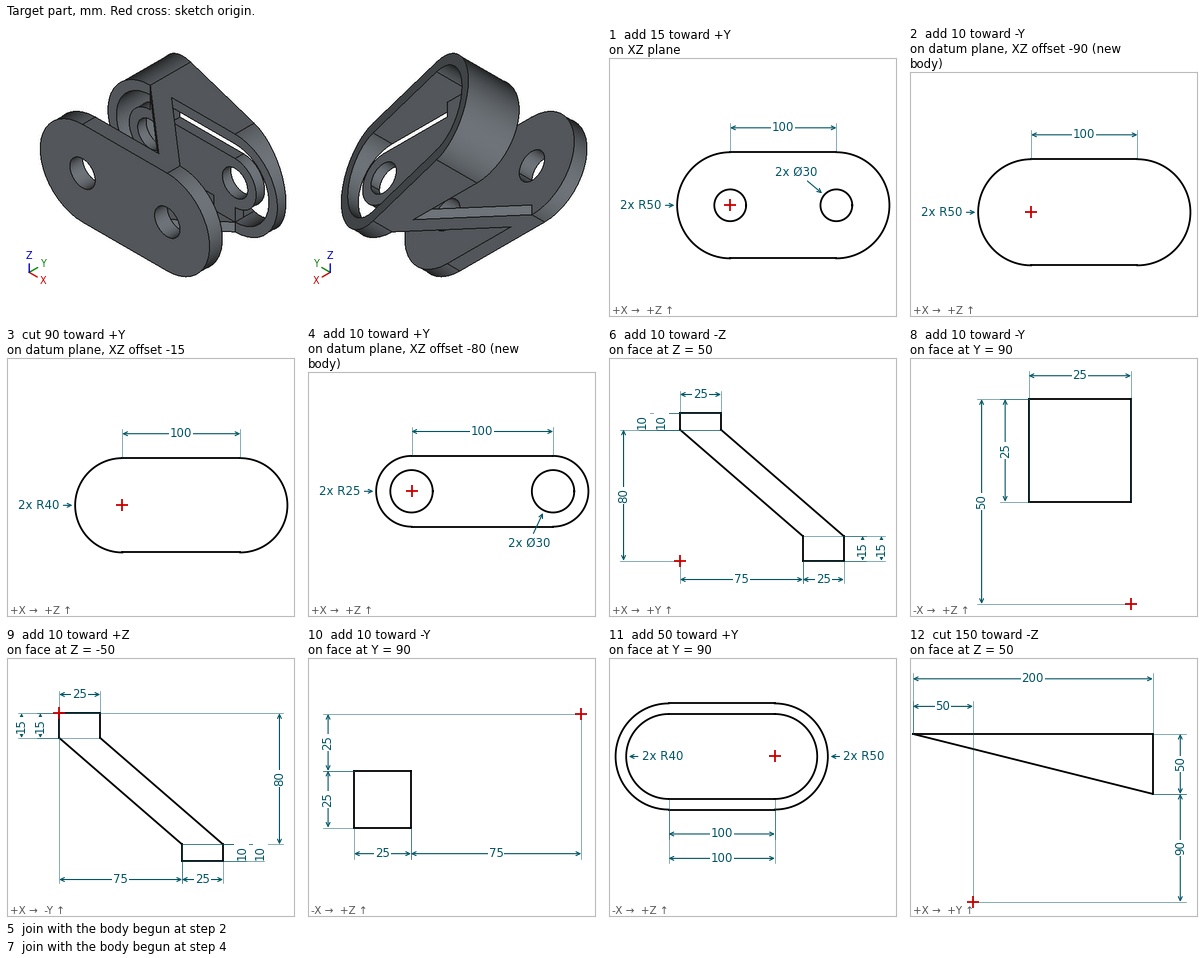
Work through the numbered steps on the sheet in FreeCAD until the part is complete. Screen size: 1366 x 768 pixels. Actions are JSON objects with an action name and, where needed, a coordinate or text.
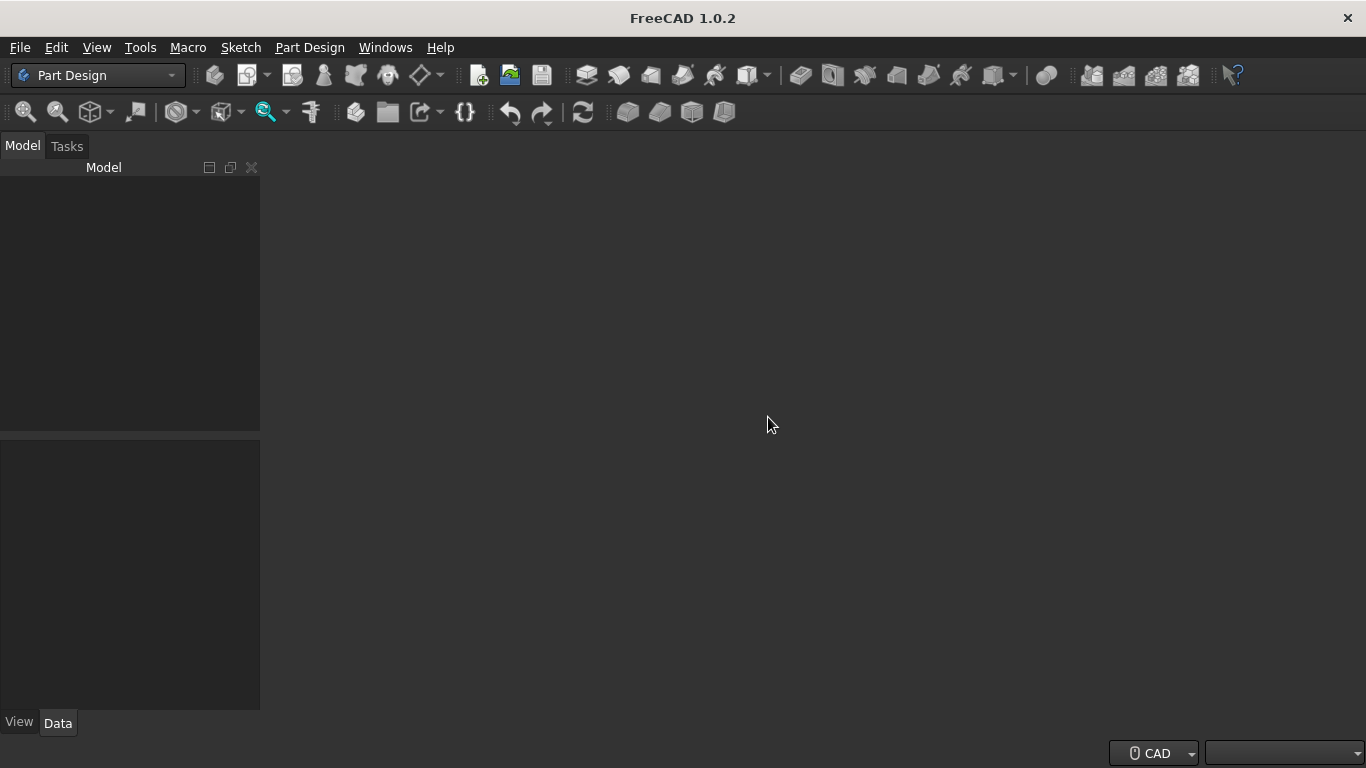
{"action": "left_click", "coordinate": [478, 76]}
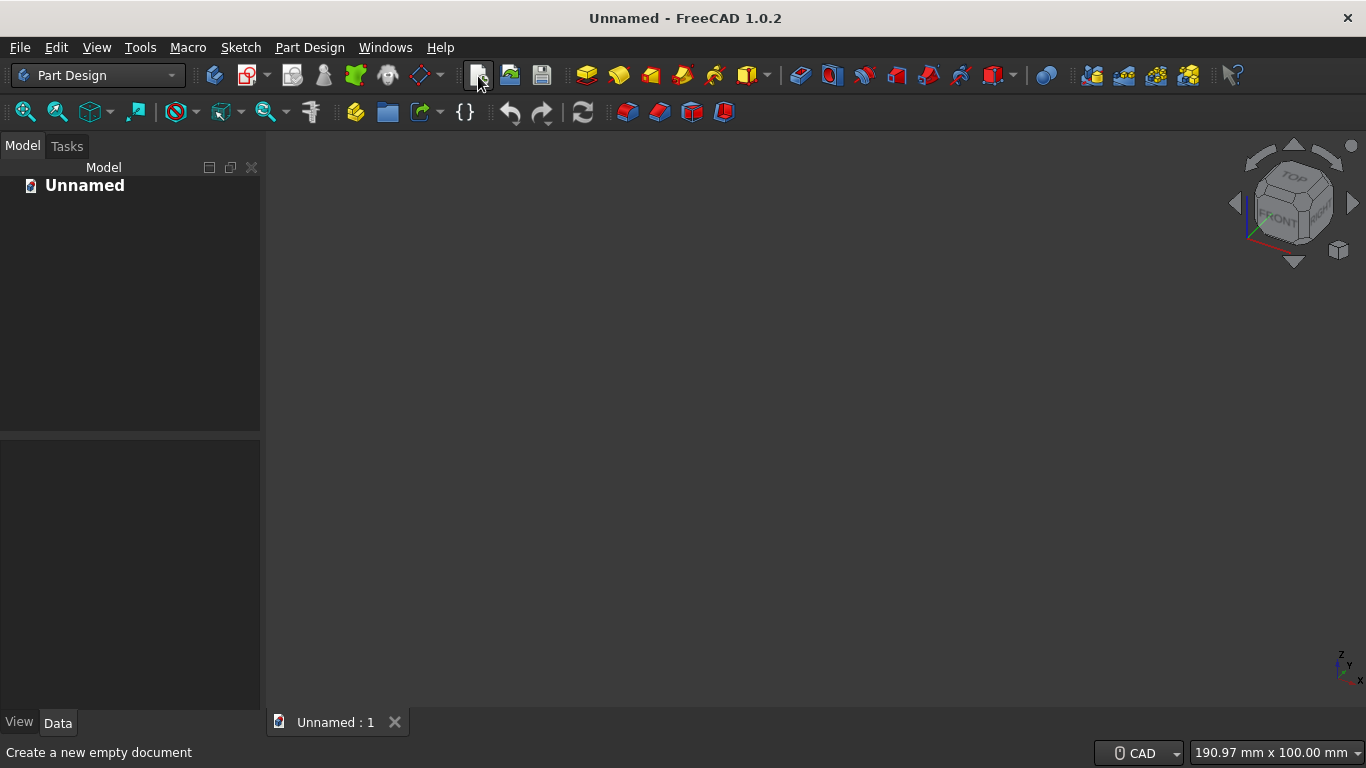
{"action": "left_click", "coordinate": [248, 76]}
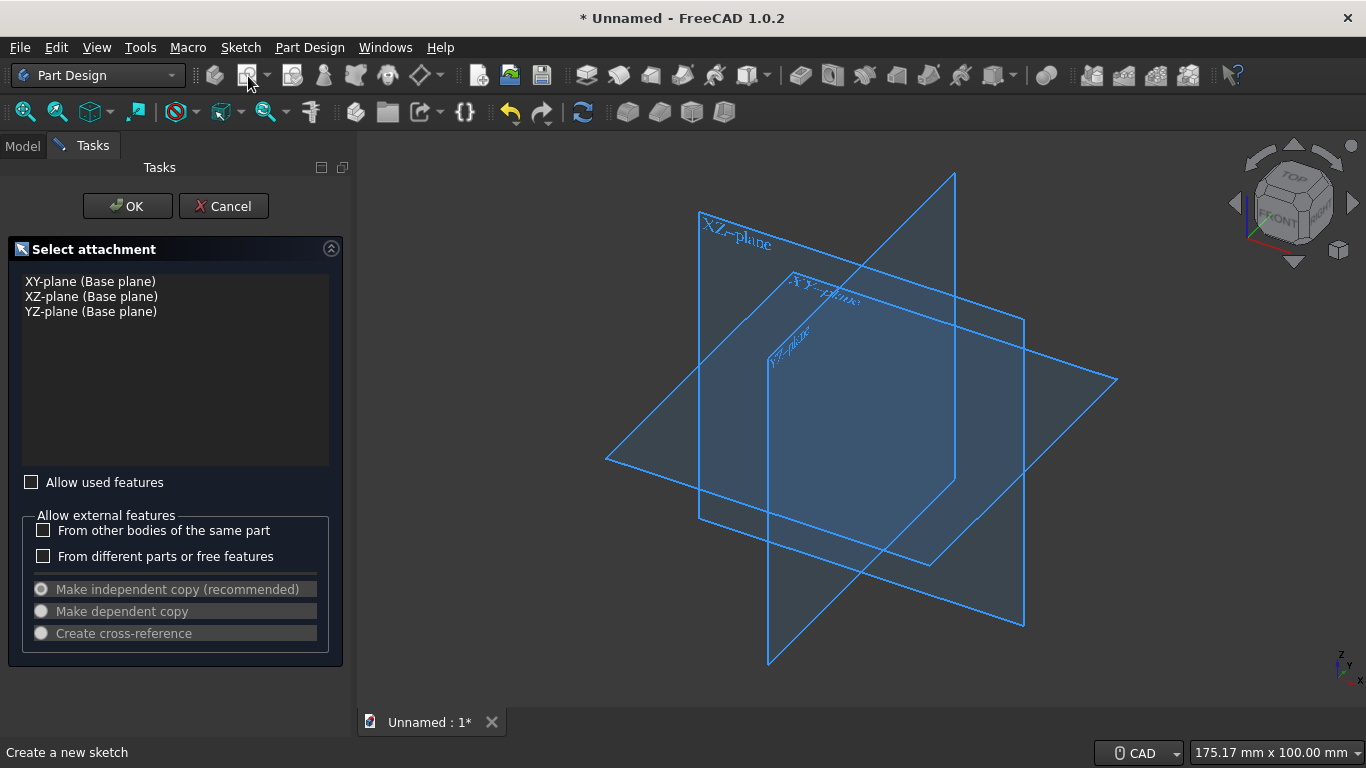
{"action": "left_click", "coordinate": [82, 296]}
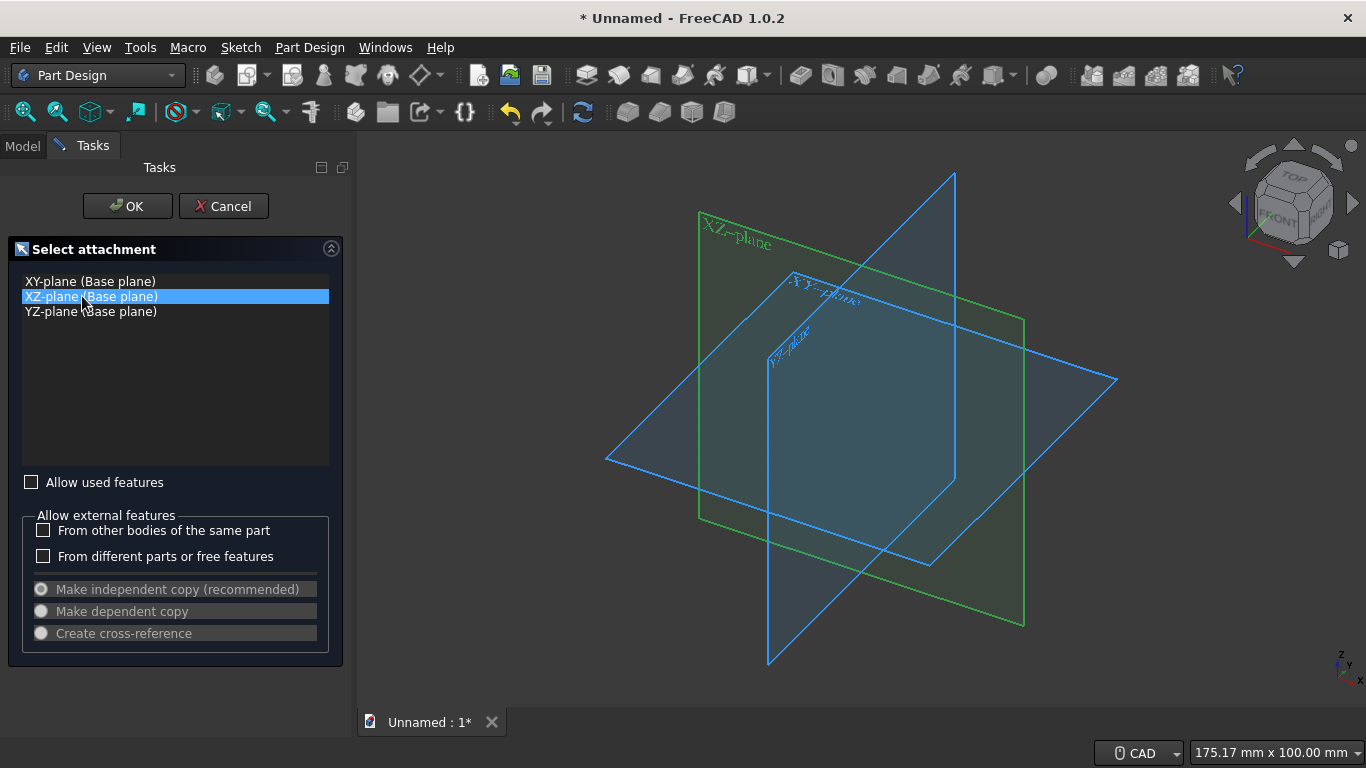
{"action": "left_click", "coordinate": [128, 206]}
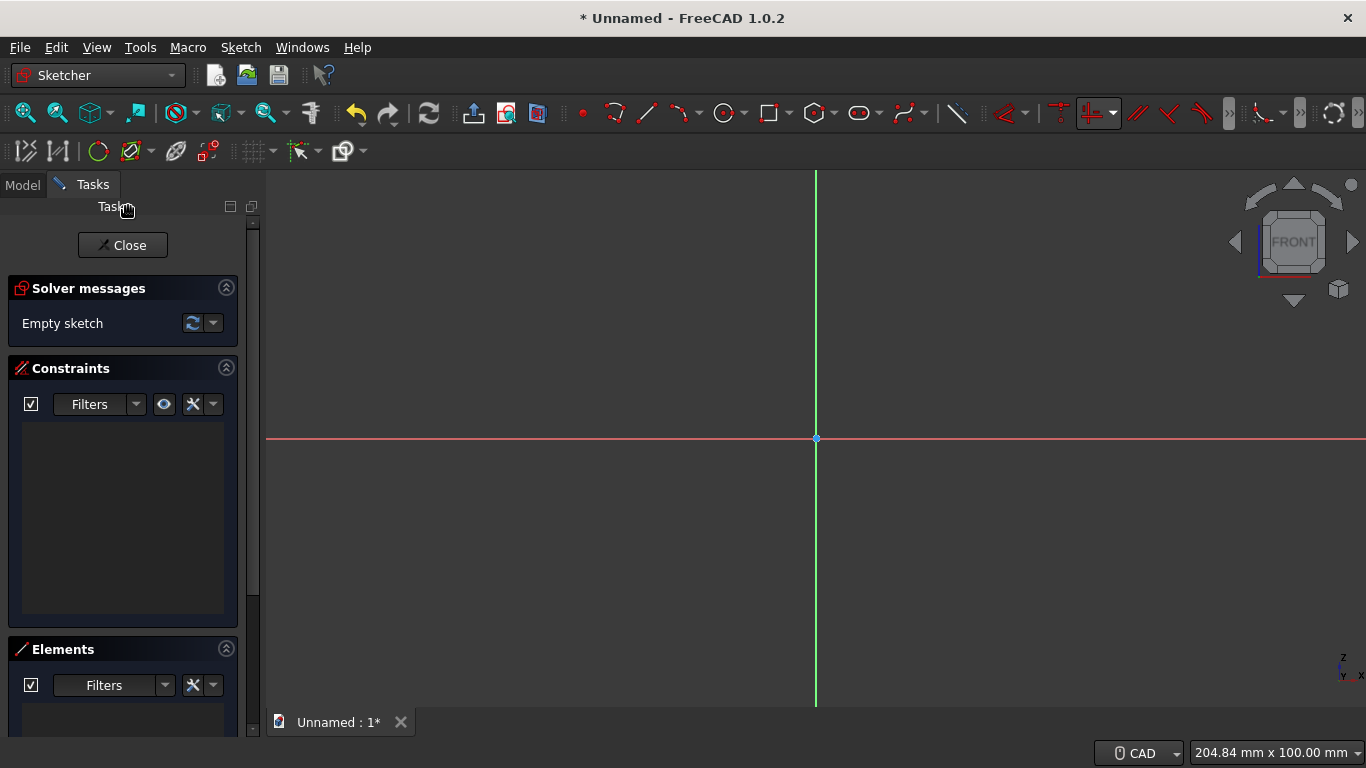
{"action": "scroll", "coordinate": [338, 438], "scroll_direction": "down", "scroll_amount": 3}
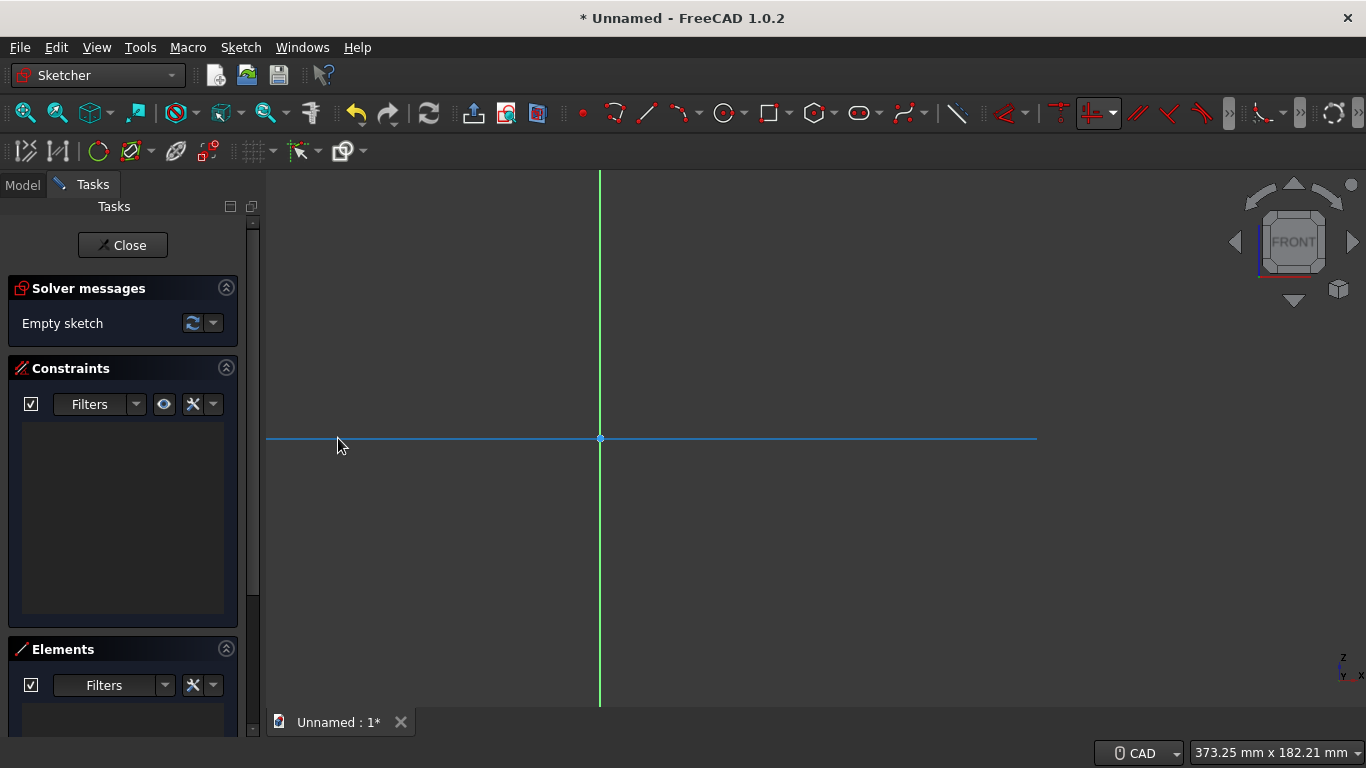
{"action": "left_click", "coordinate": [860, 114]}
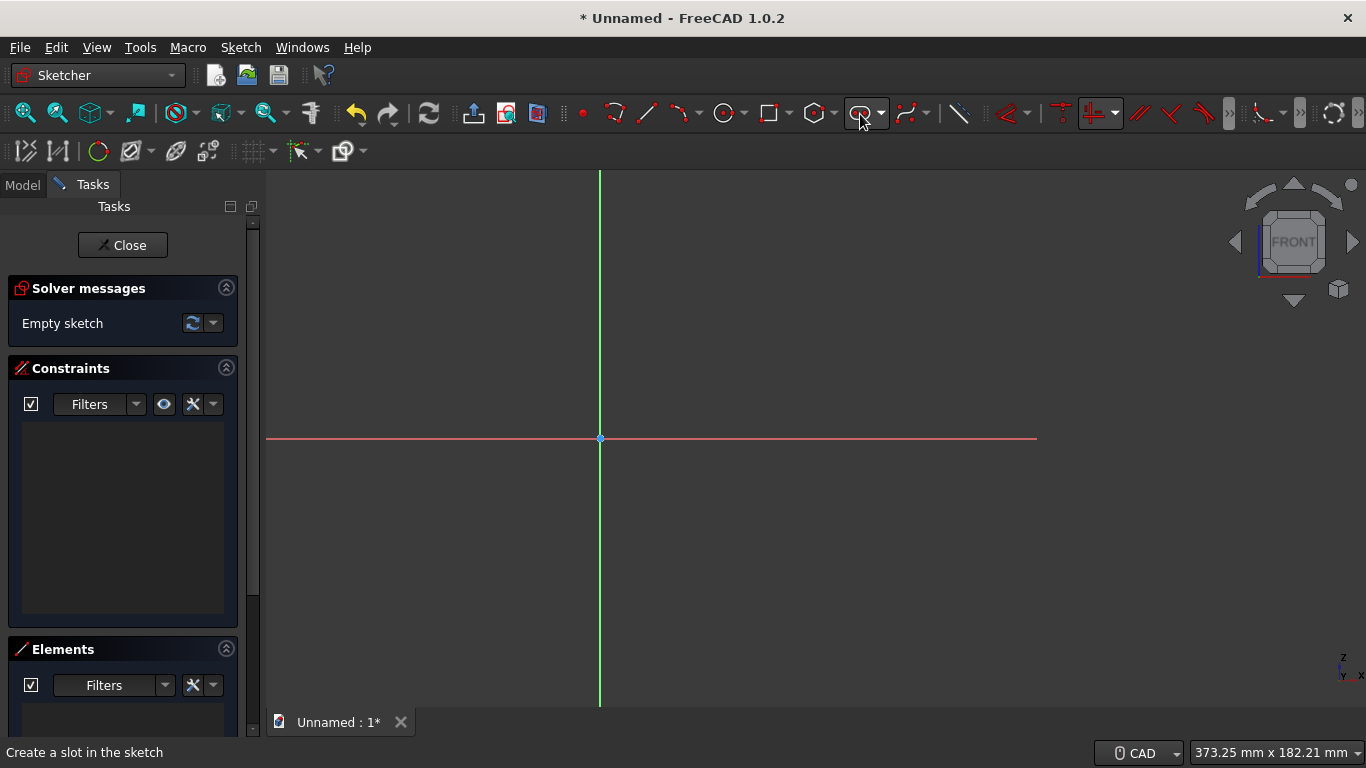
{"action": "left_click", "coordinate": [600, 438]}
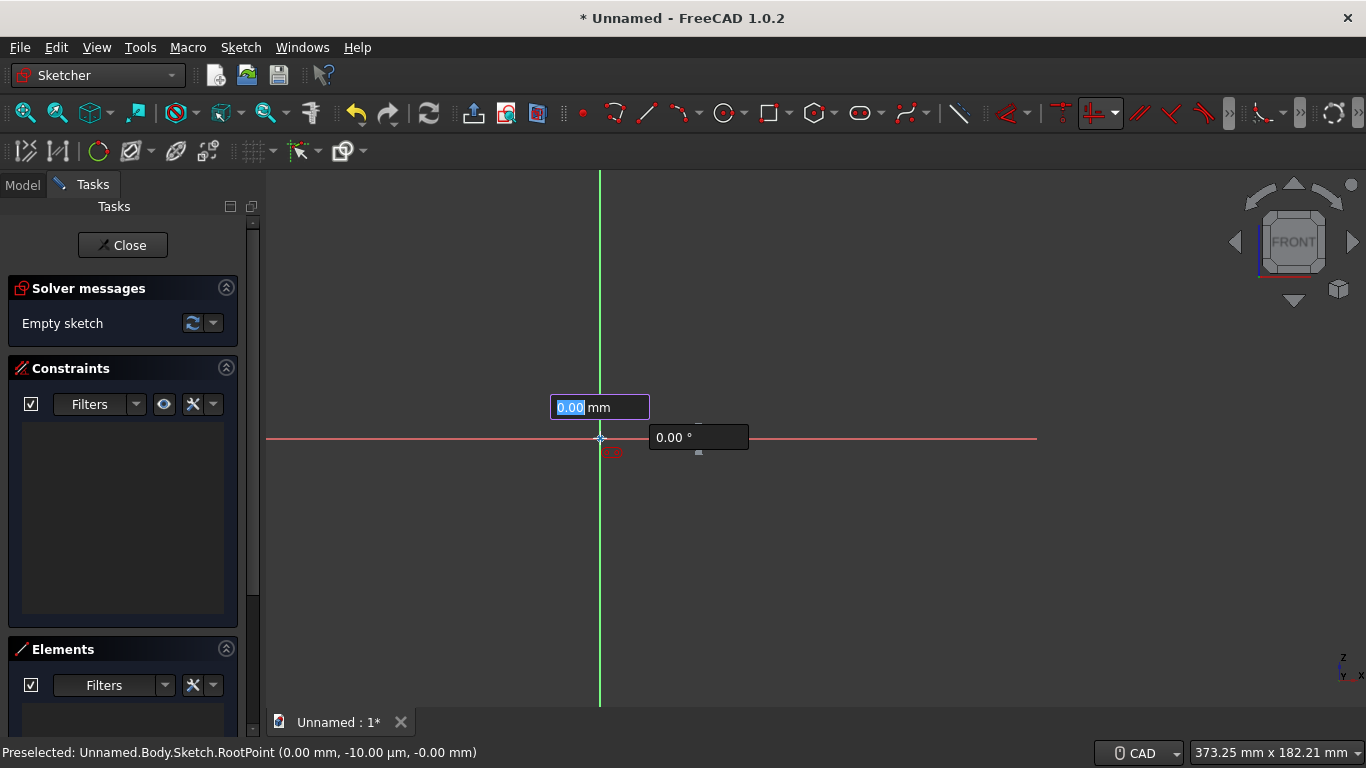
{"action": "left_click", "coordinate": [895, 430]}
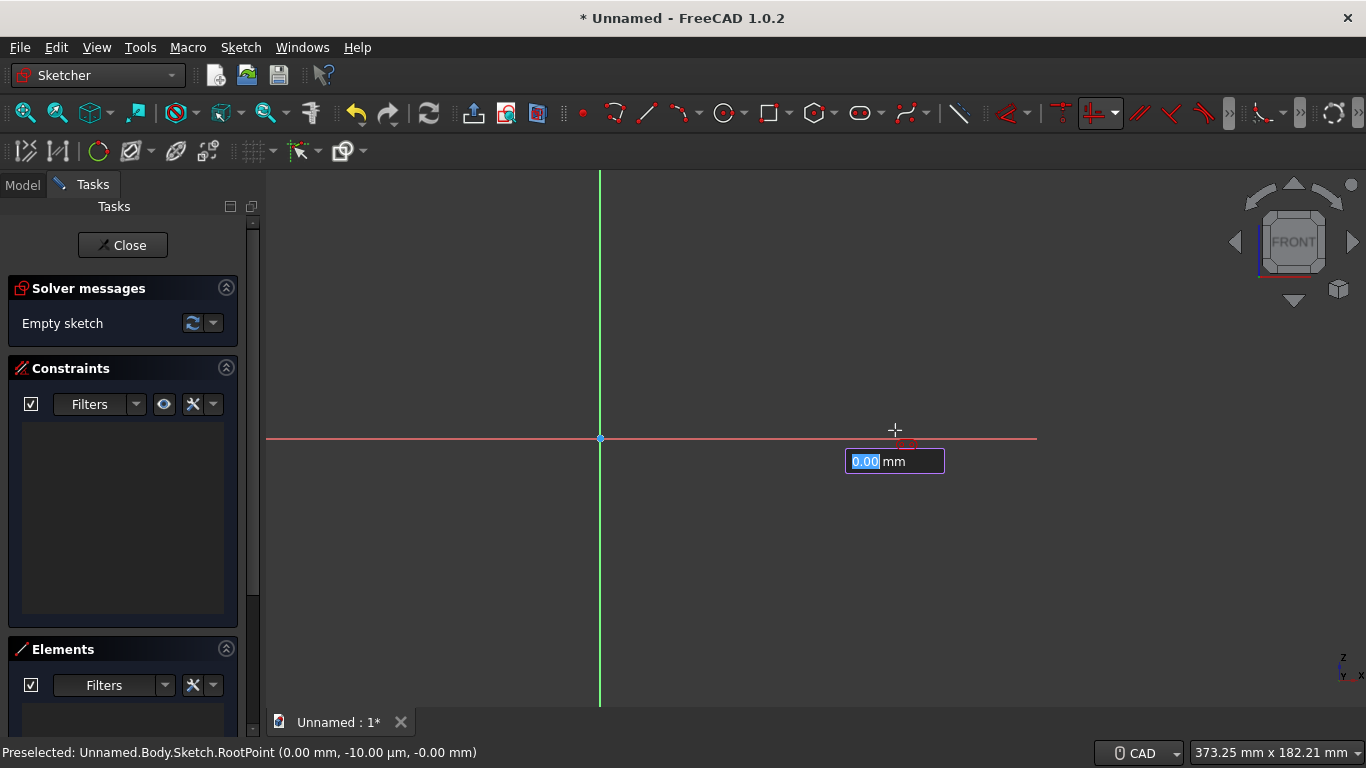
{"action": "left_click", "coordinate": [748, 586]}